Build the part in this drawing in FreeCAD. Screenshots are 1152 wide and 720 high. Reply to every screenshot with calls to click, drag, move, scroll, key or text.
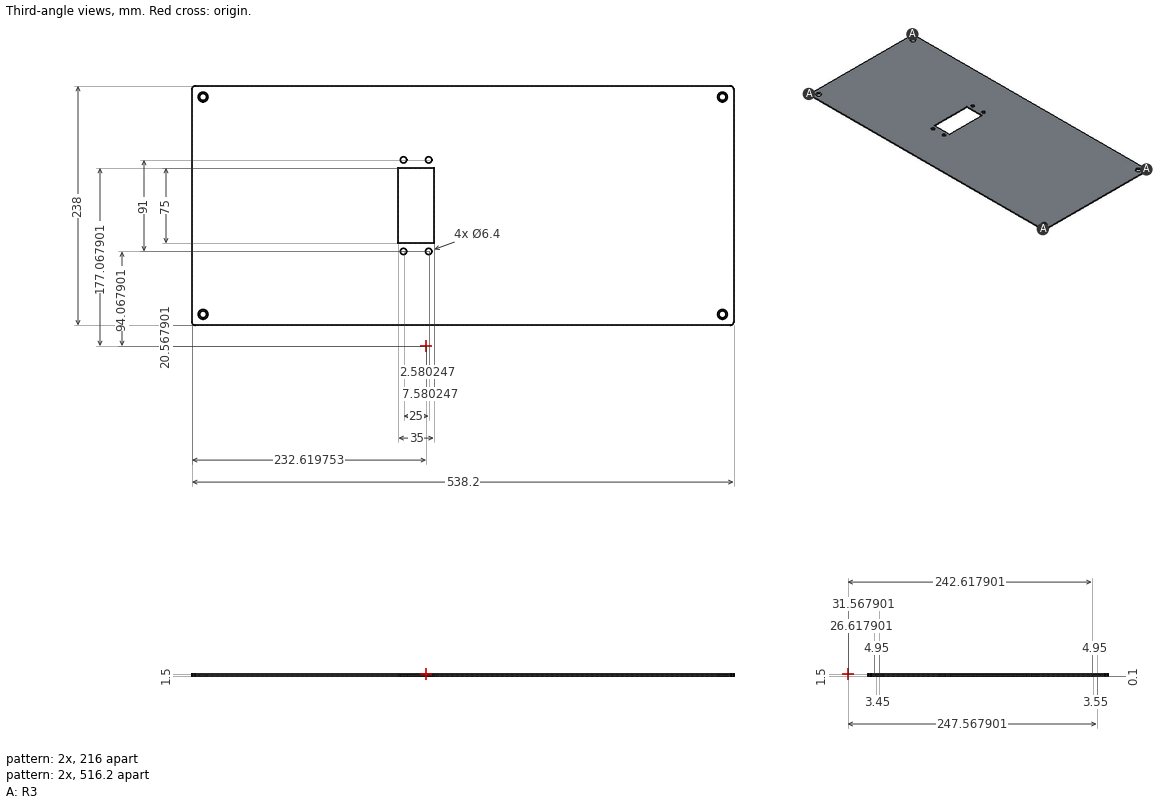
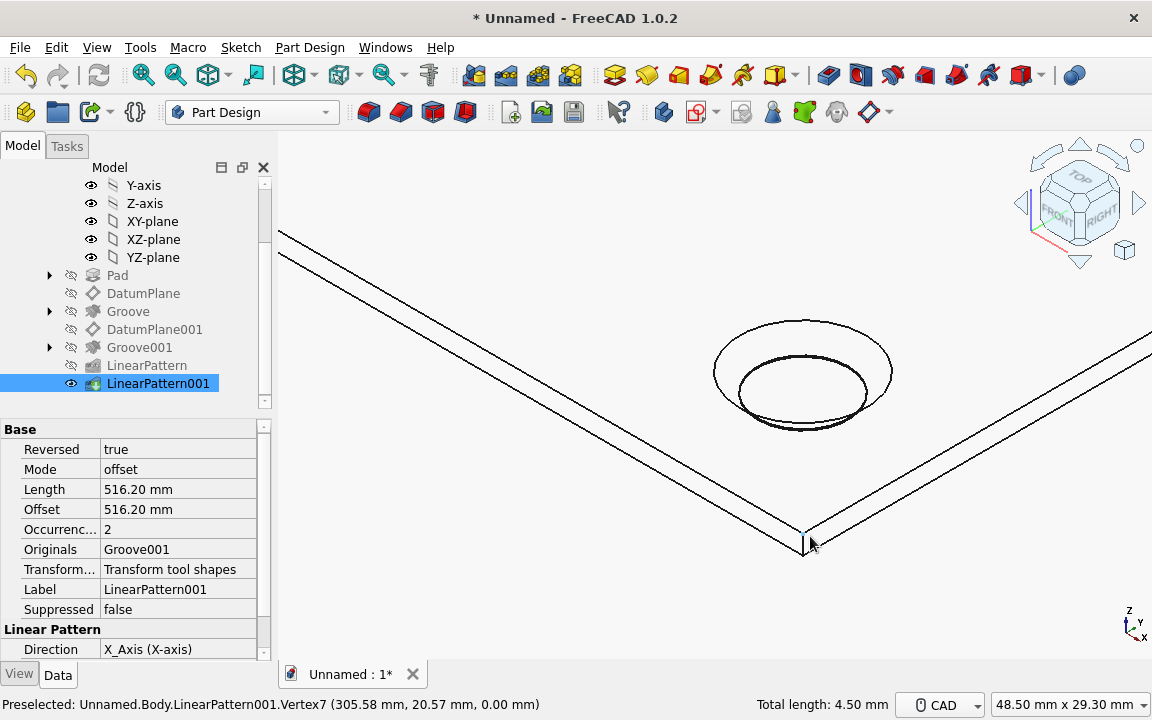
click(803, 544, ctrl)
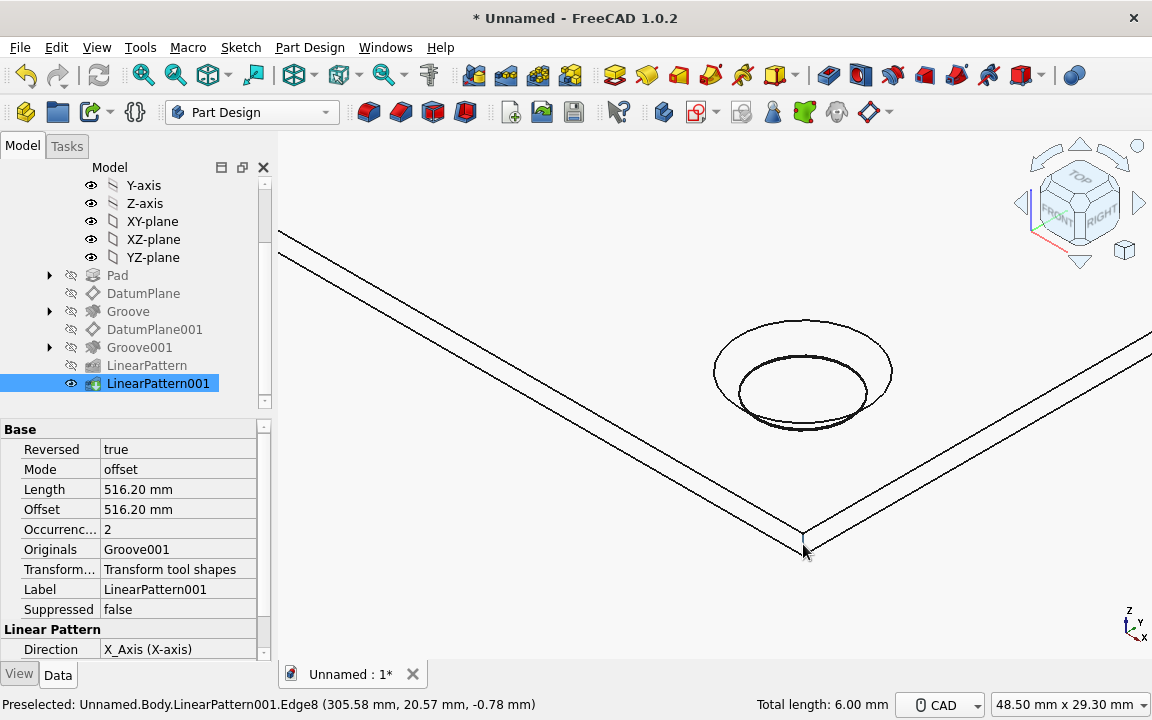
key(v)
key(1)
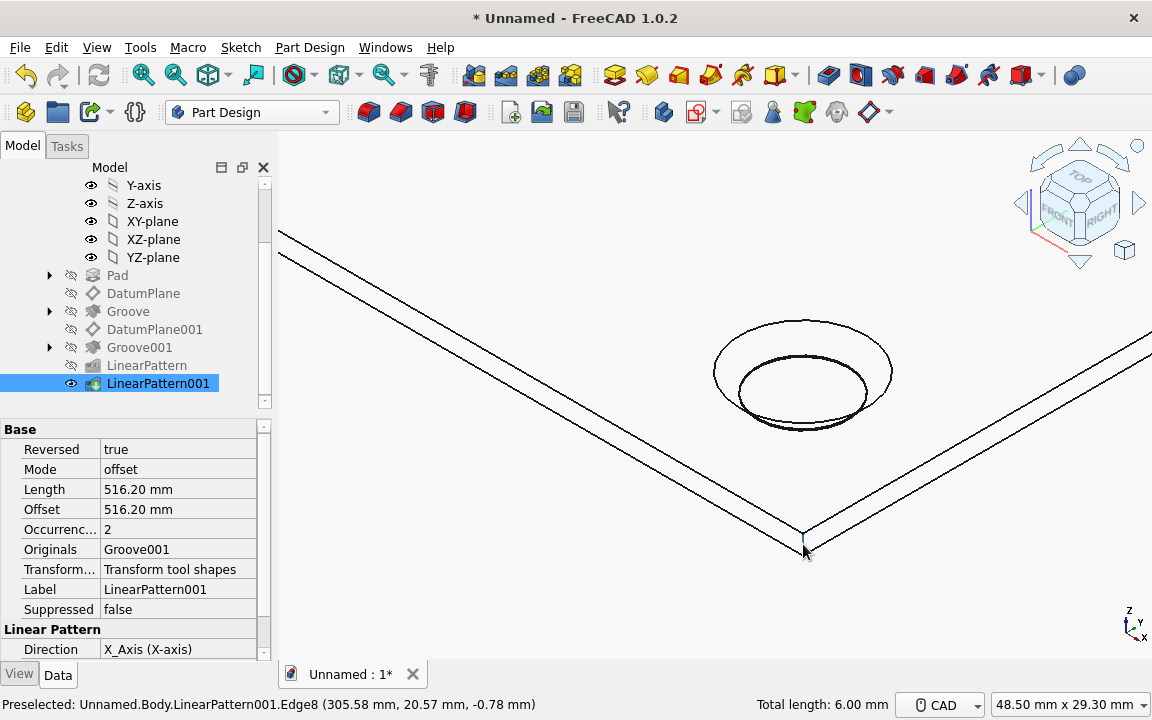
click(370, 112)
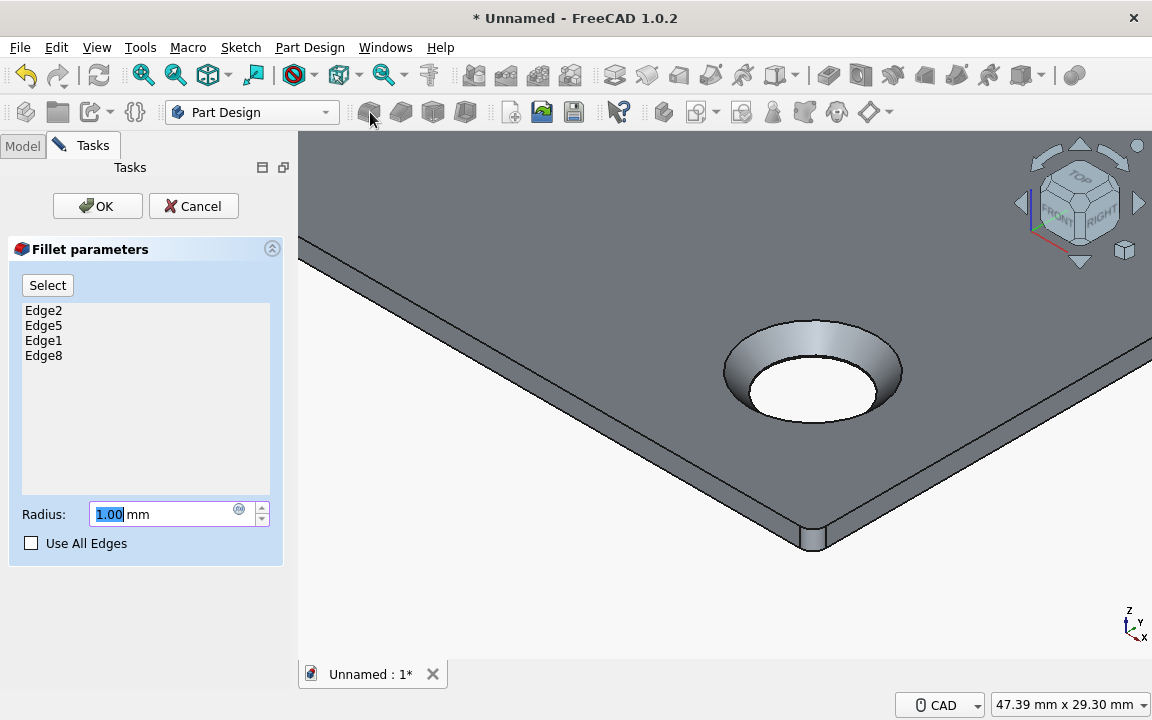
text(3)
key(Tab)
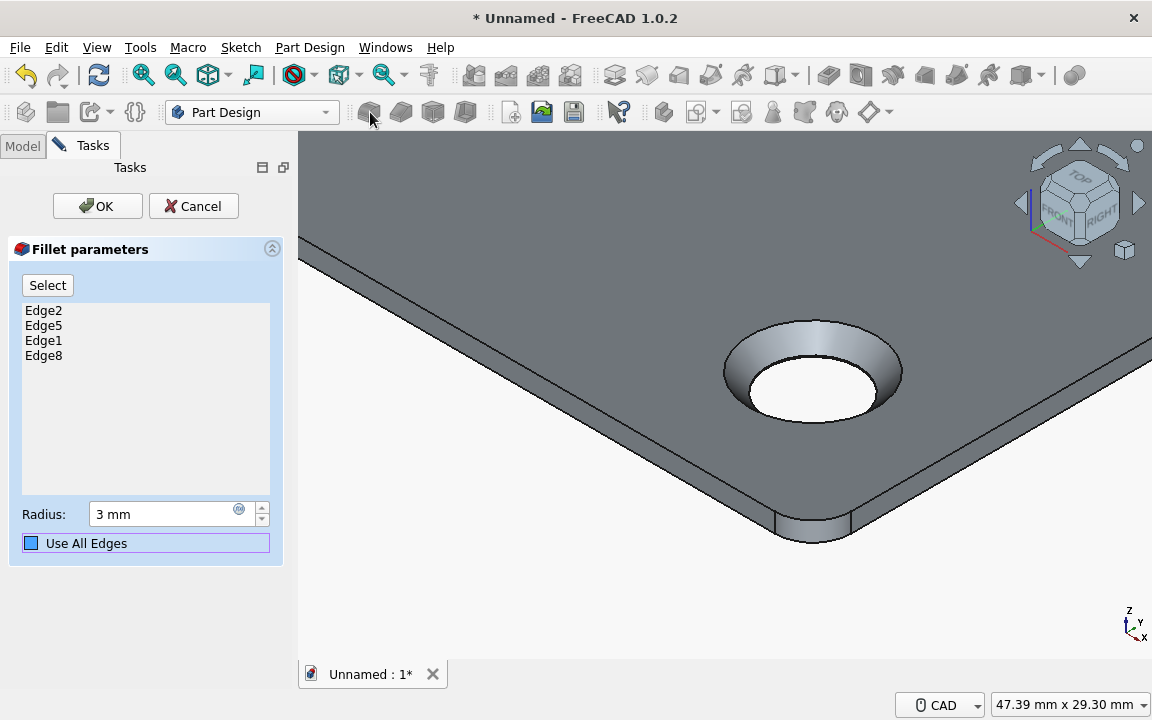
click(98, 206)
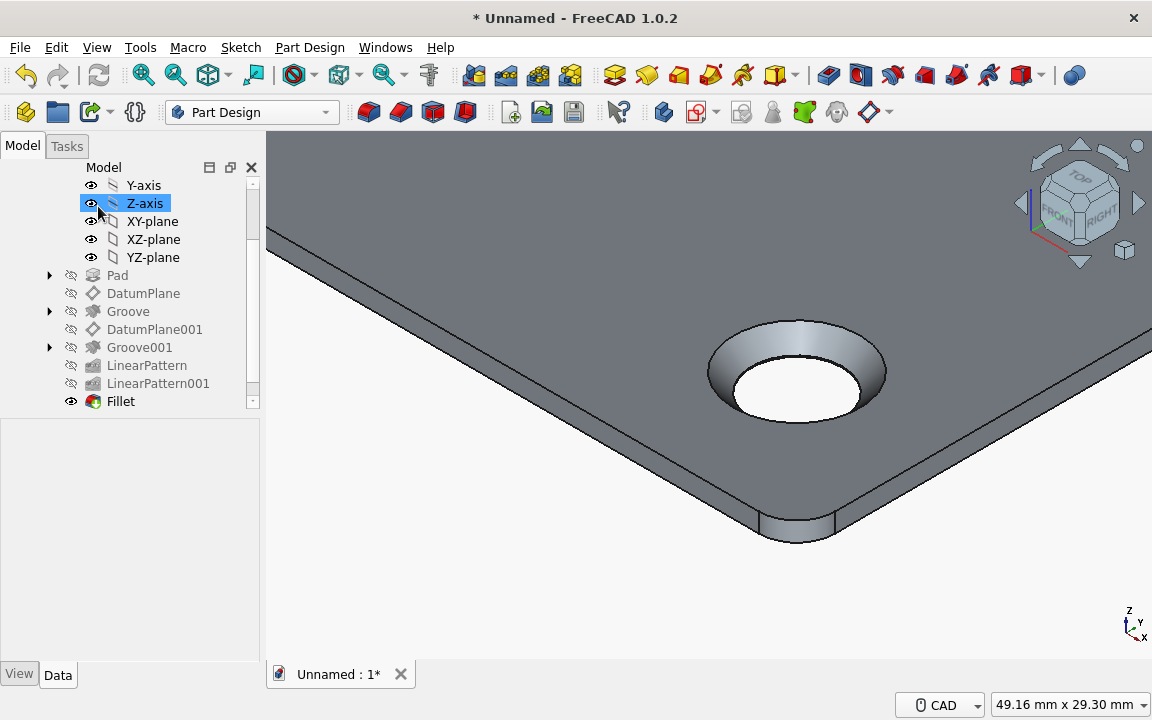
click(144, 76)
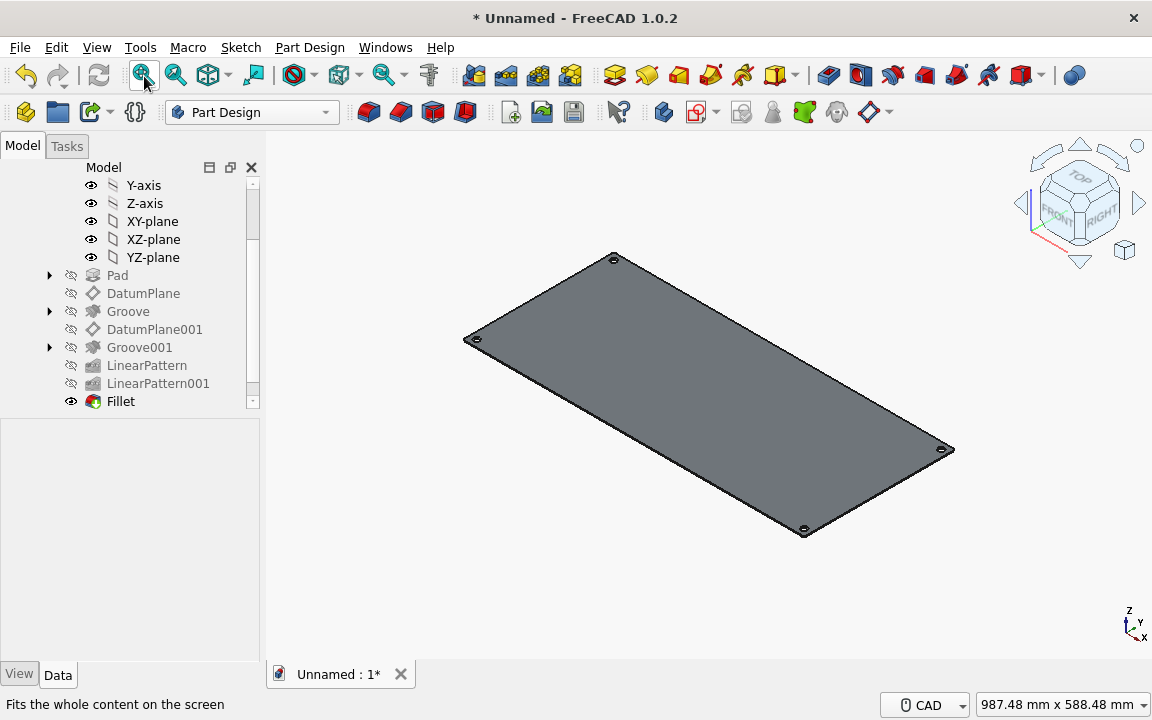
click(758, 422)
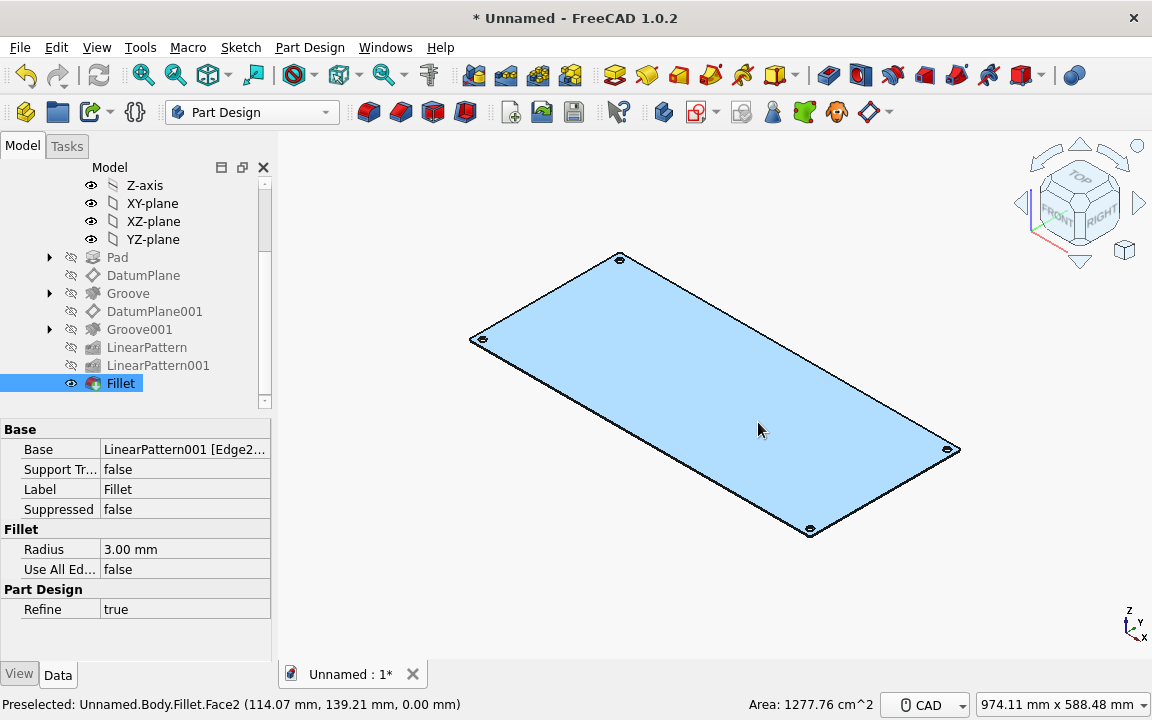
click(696, 112)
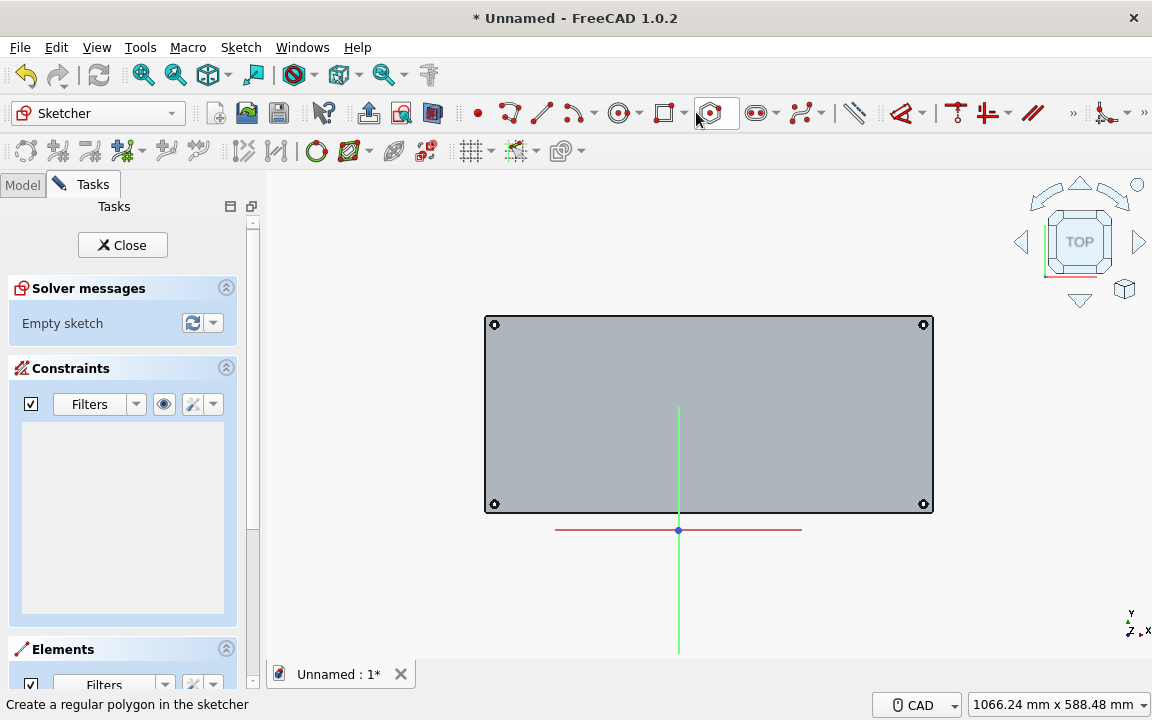
scroll(695, 492, up, 4)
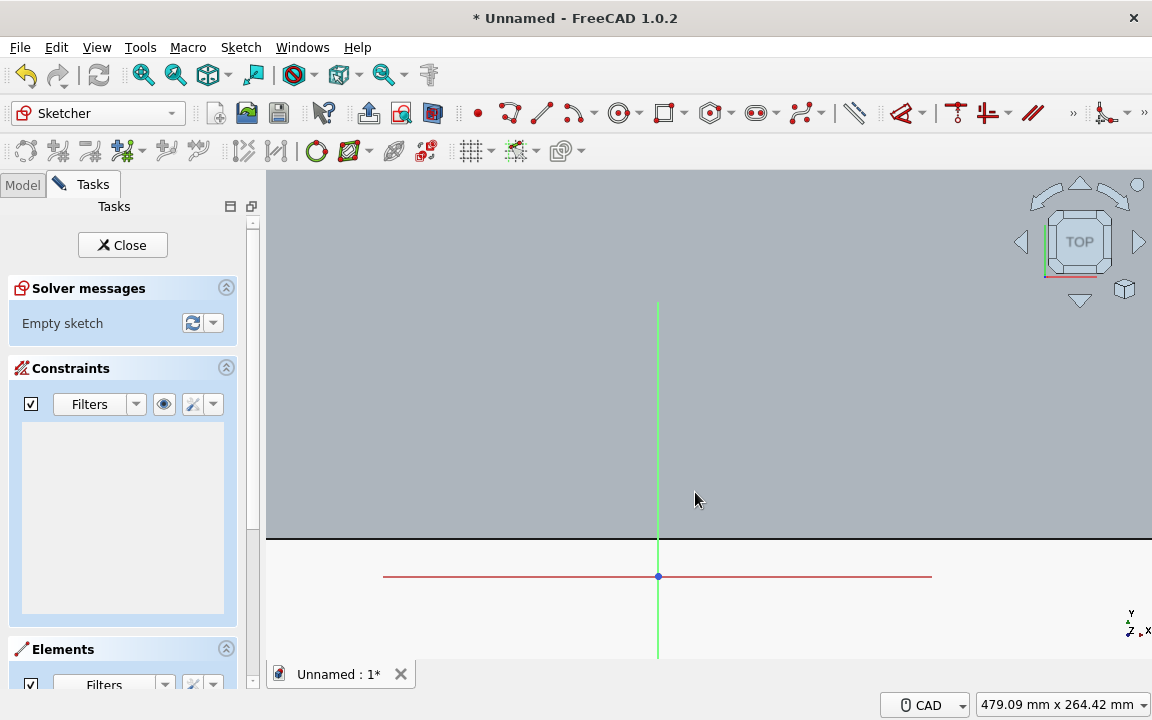
click(664, 114)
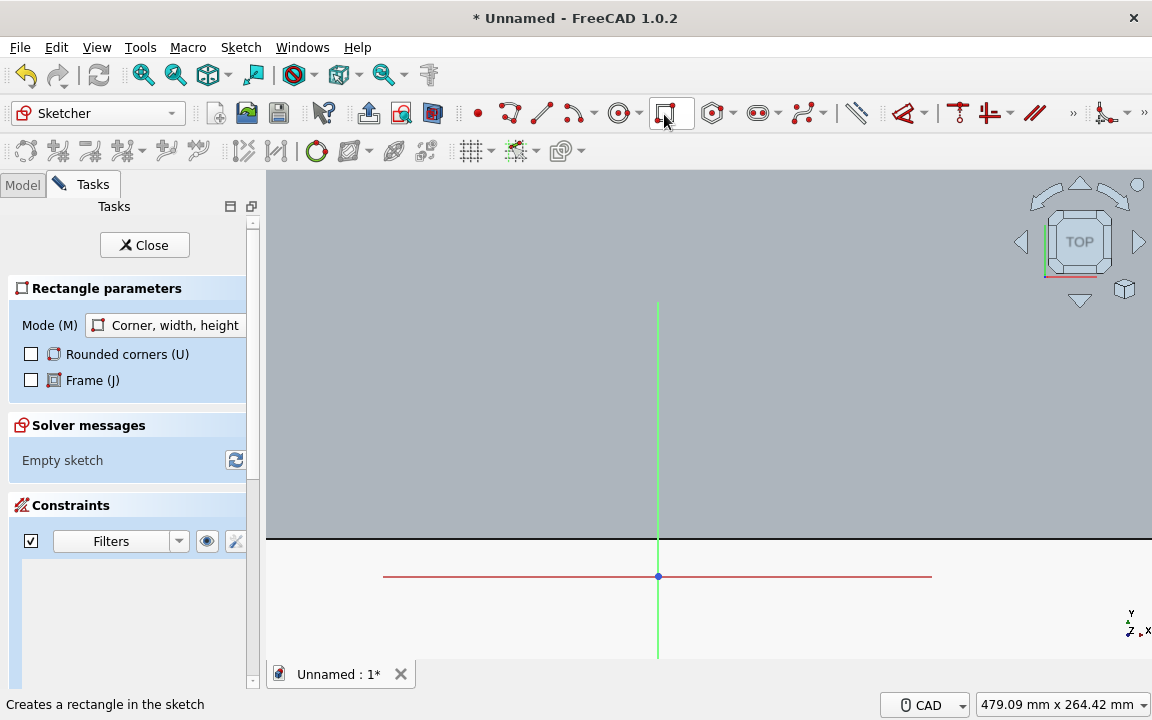
click(607, 249)
click(672, 388)
key(Escape)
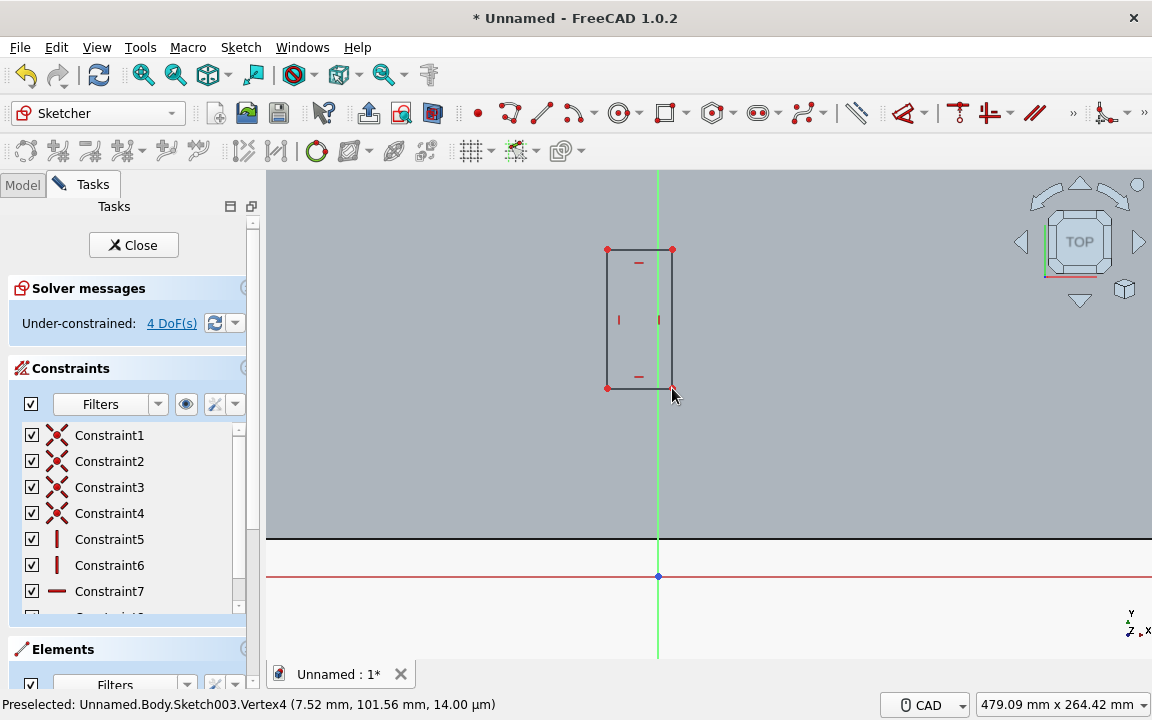
click(904, 114)